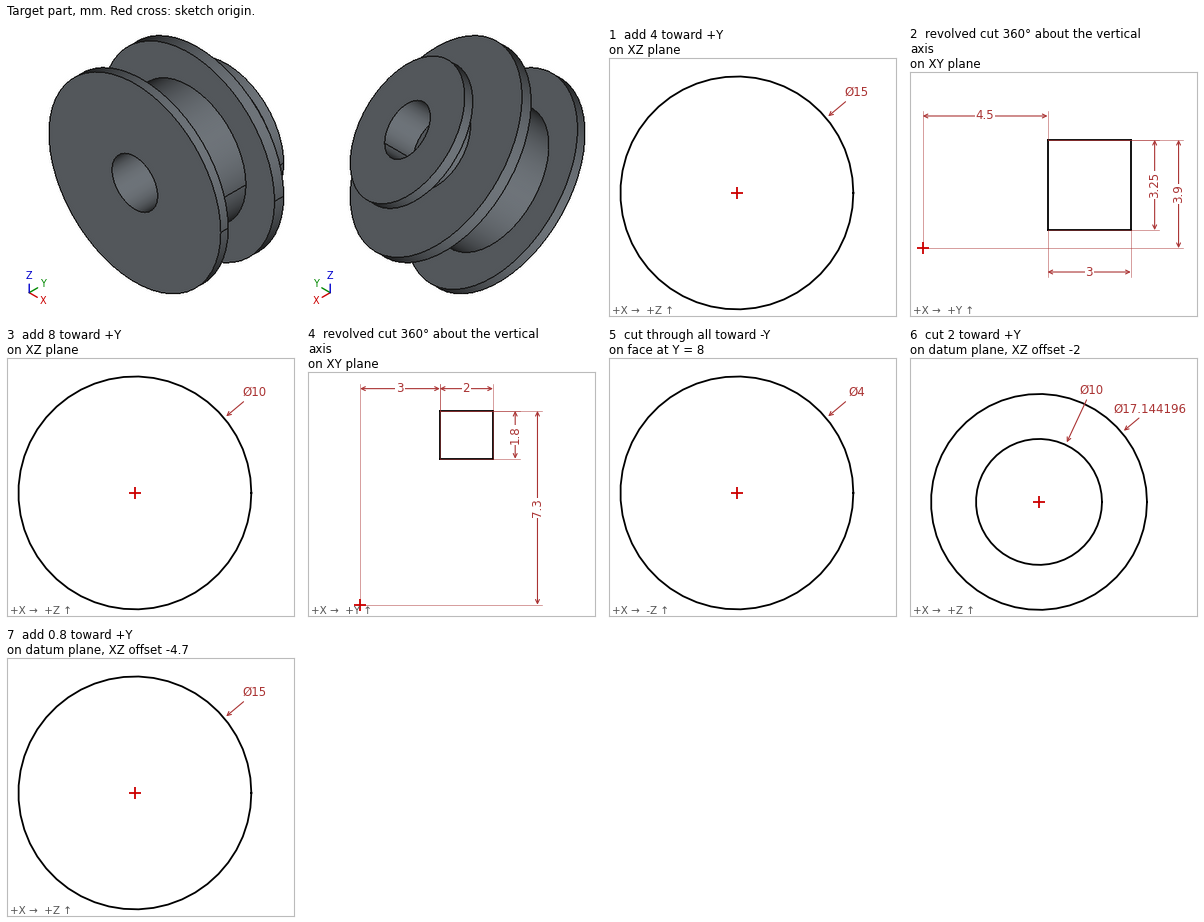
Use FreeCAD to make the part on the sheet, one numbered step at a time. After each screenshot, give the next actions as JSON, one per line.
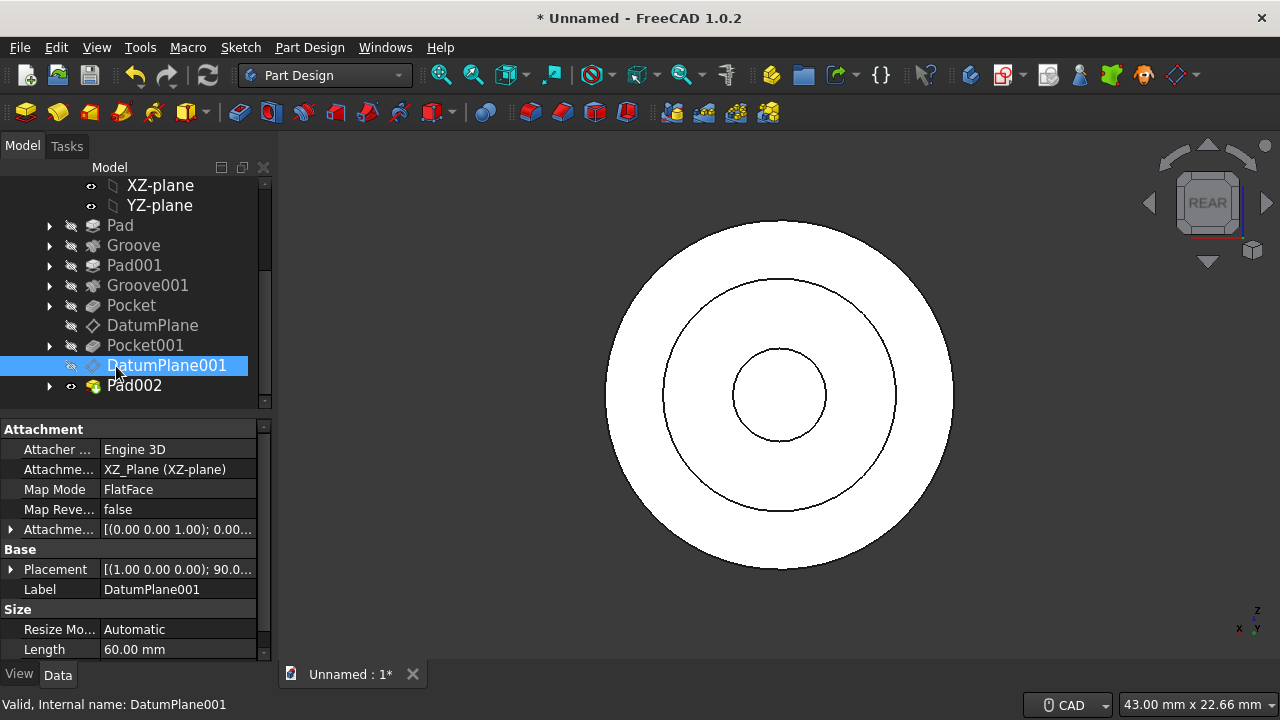
{"action": "key", "text": "0"}